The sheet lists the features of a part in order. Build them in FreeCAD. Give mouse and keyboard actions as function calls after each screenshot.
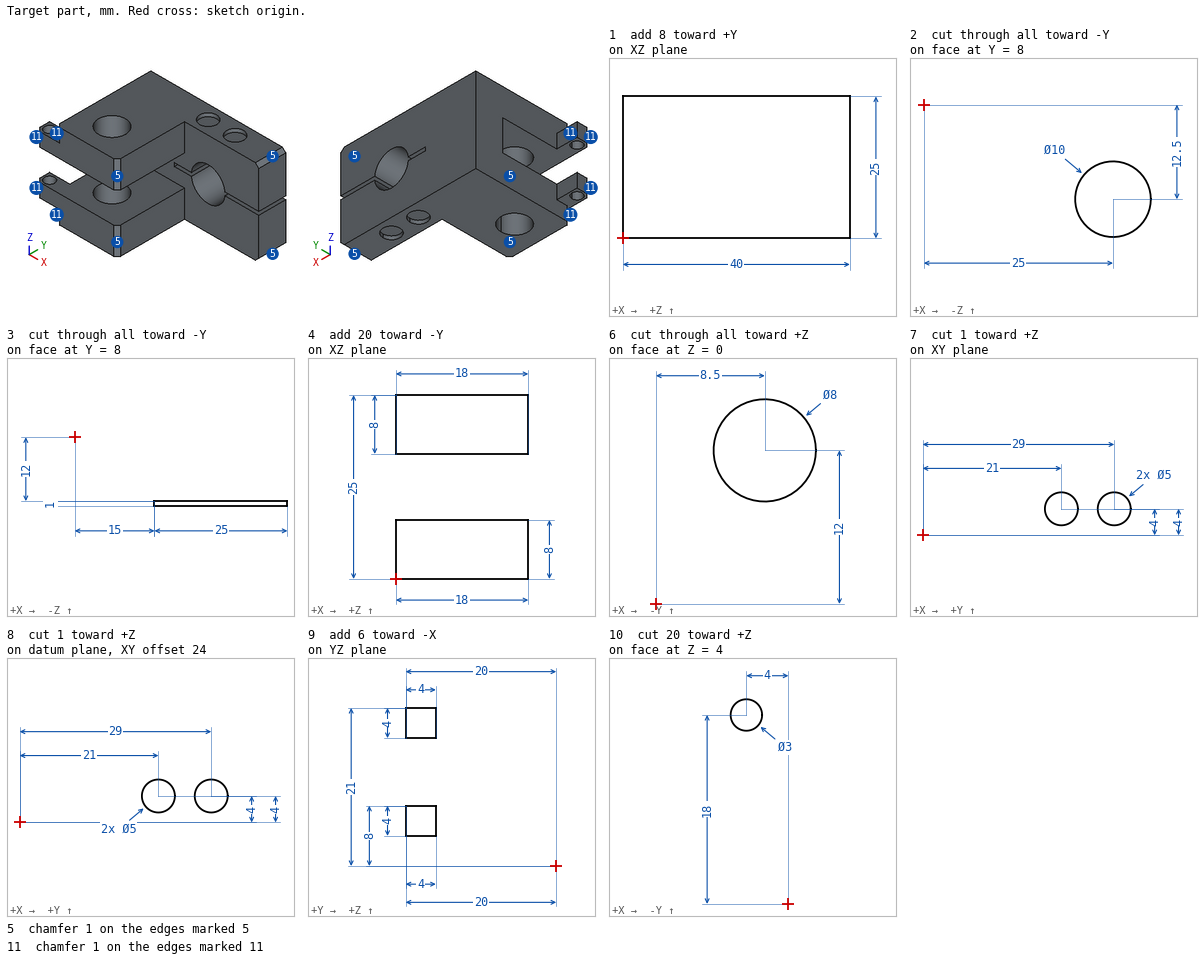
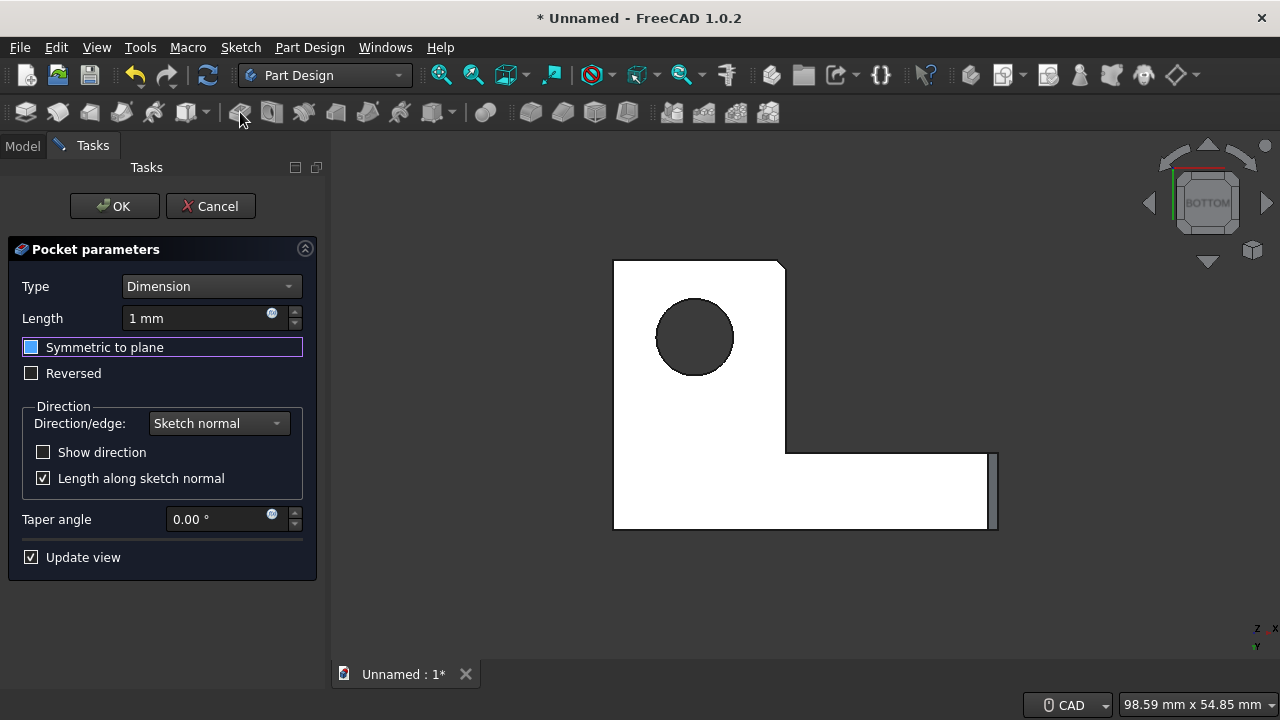
click(30, 373)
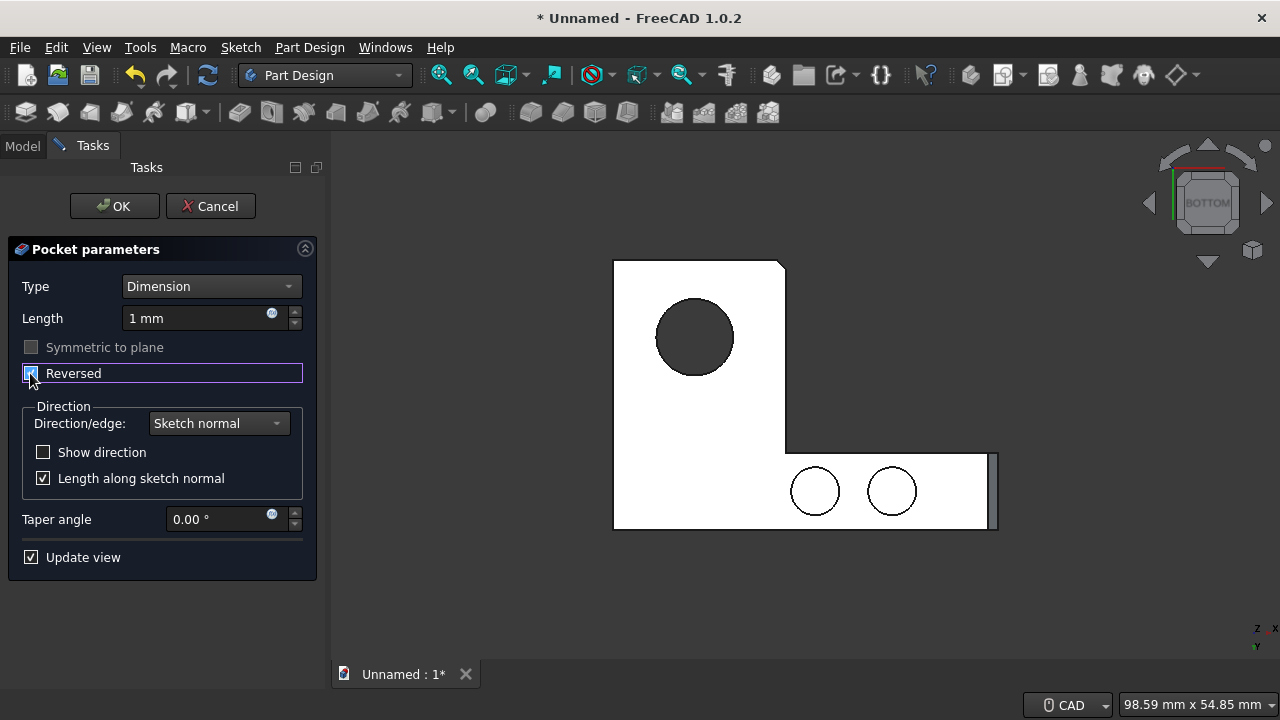
click(115, 206)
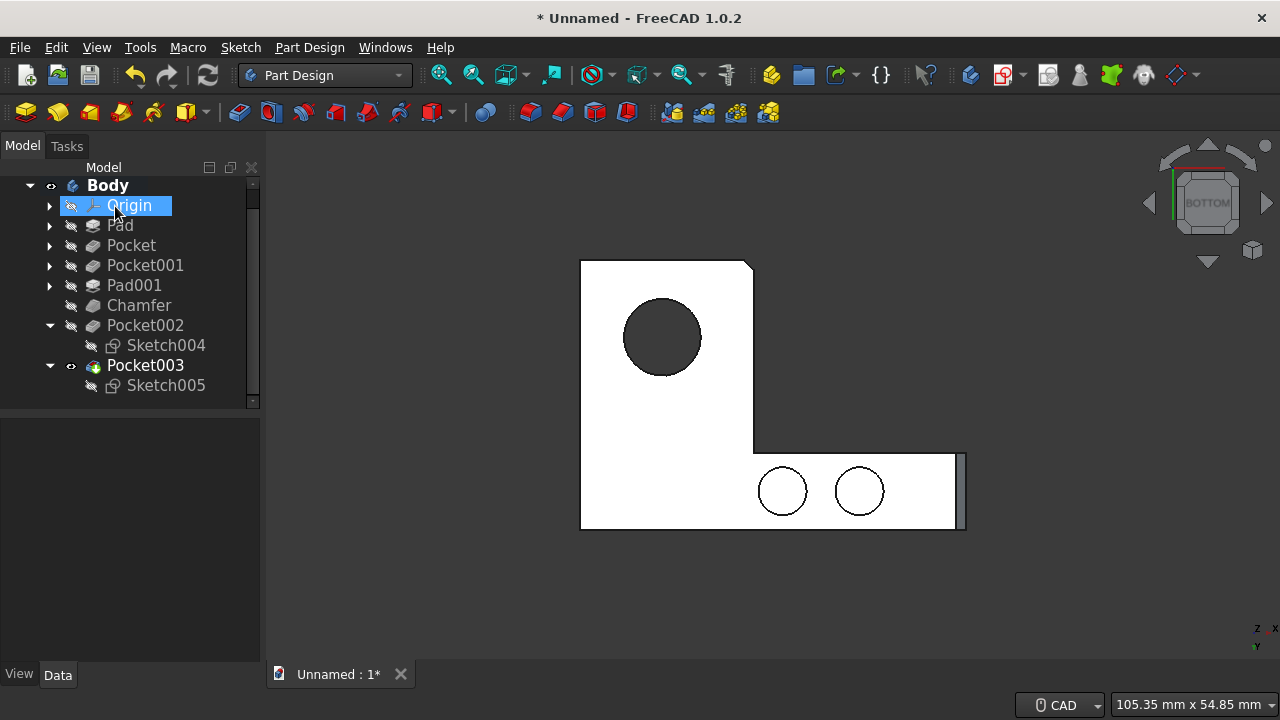
click(50, 206)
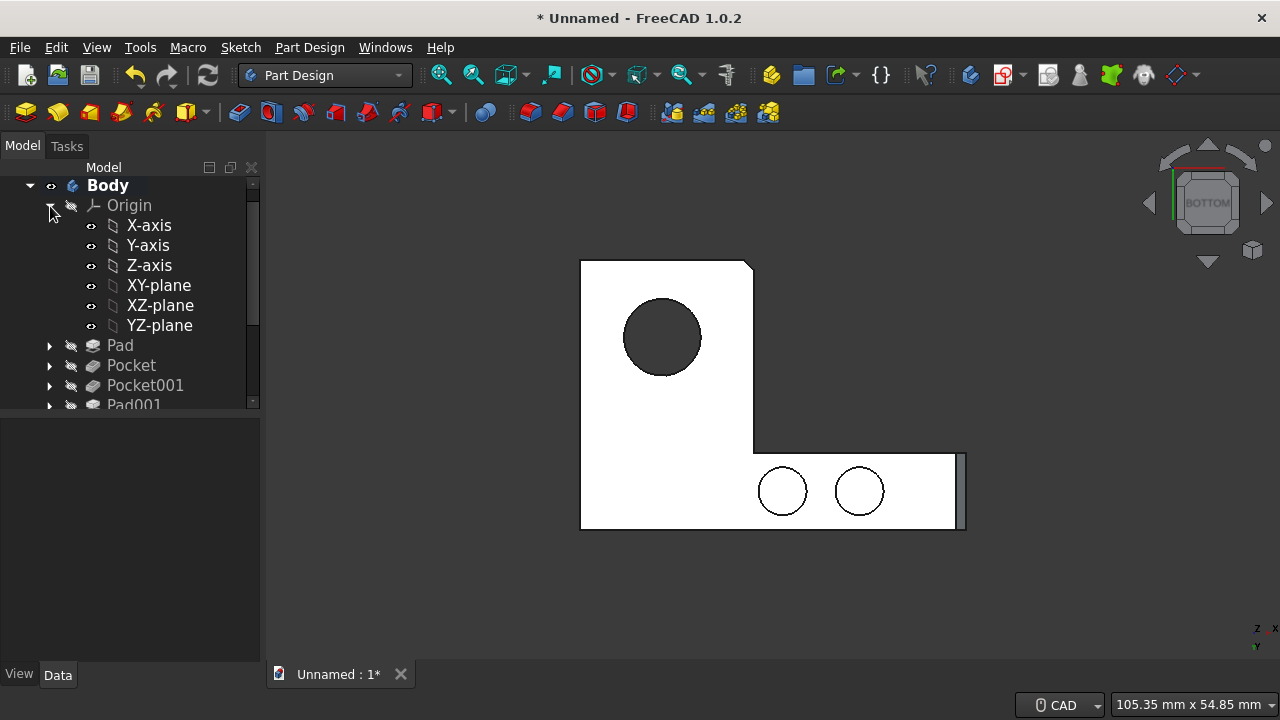
click(136, 286)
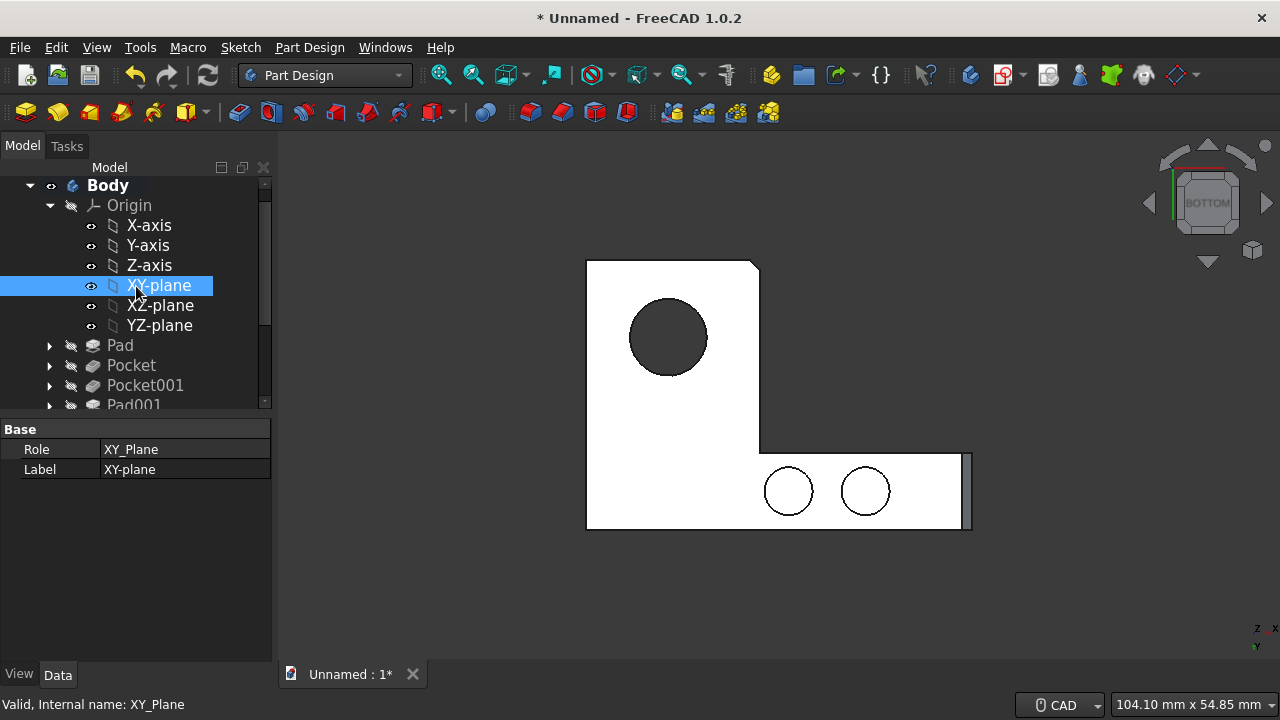
click(1176, 76)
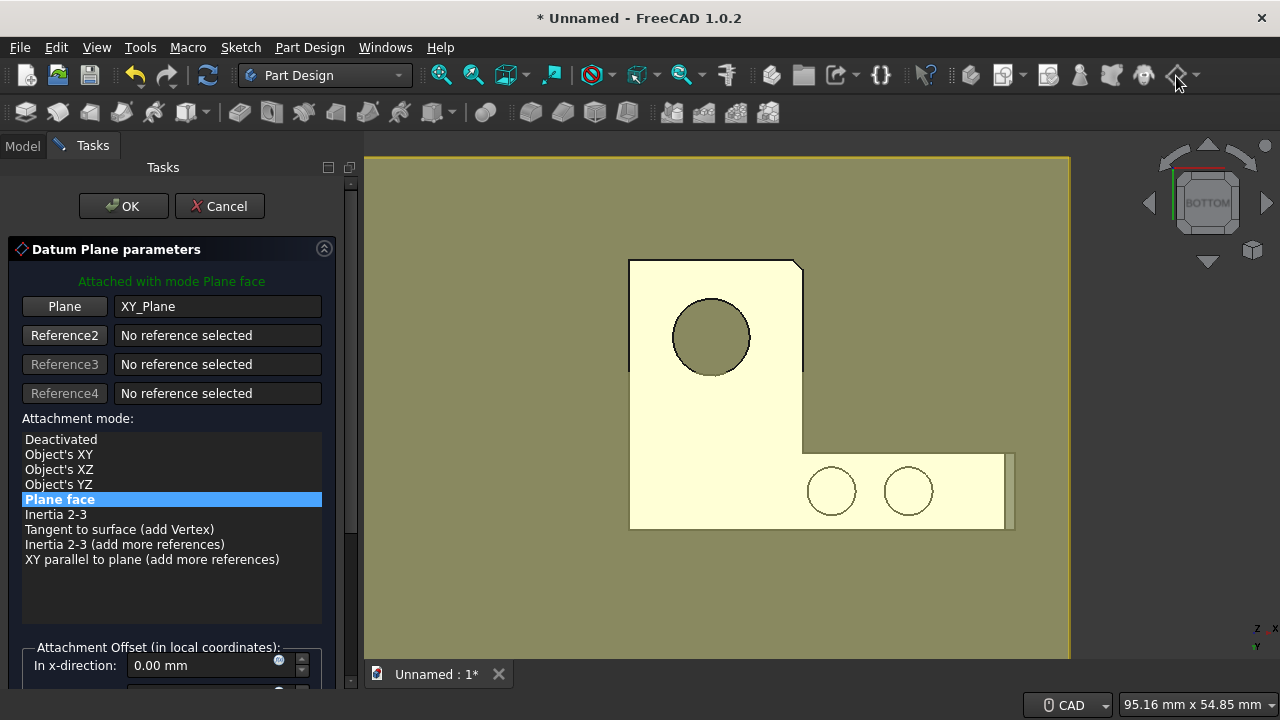
scroll(351, 432, down, 2)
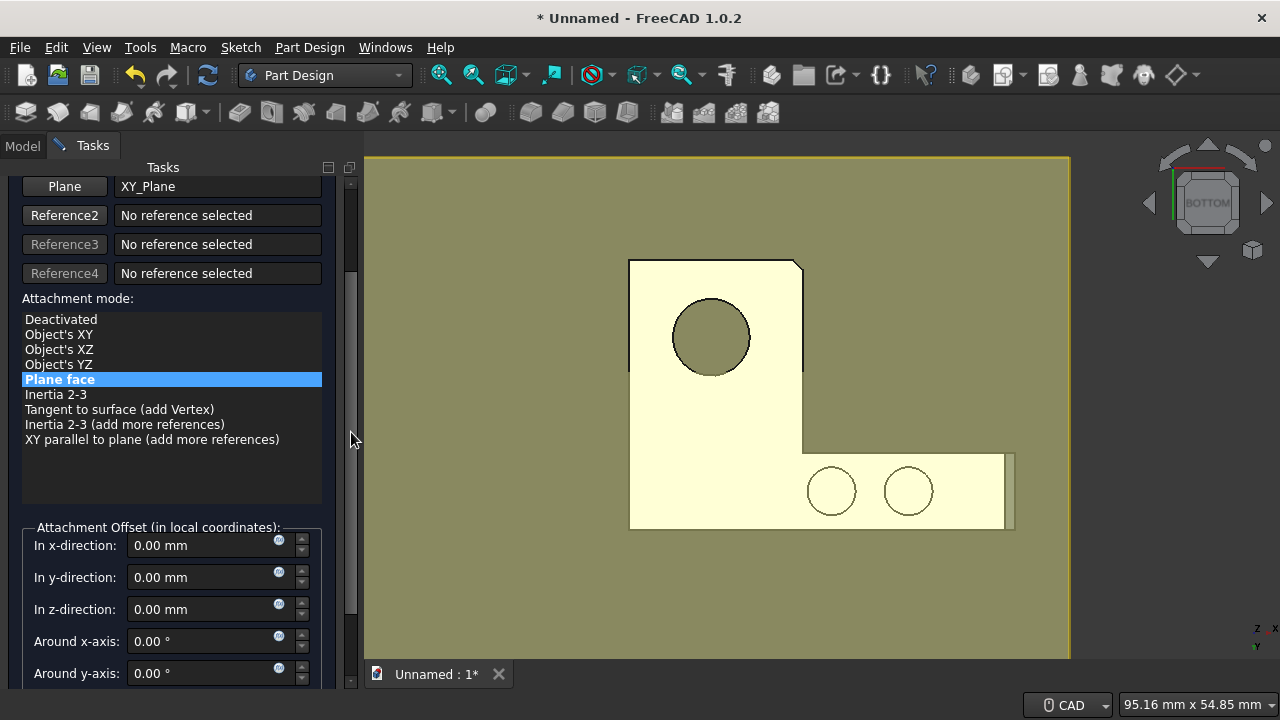
triple_click(210, 609)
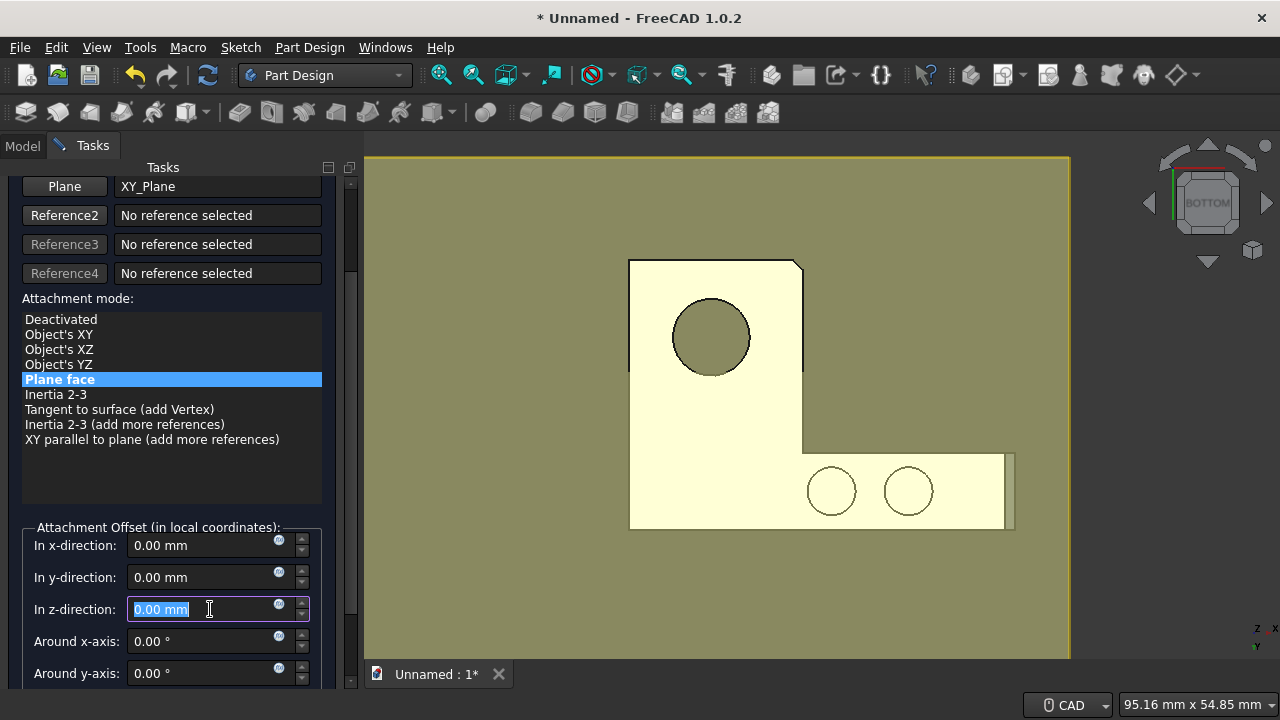
text(24)
key(Tab)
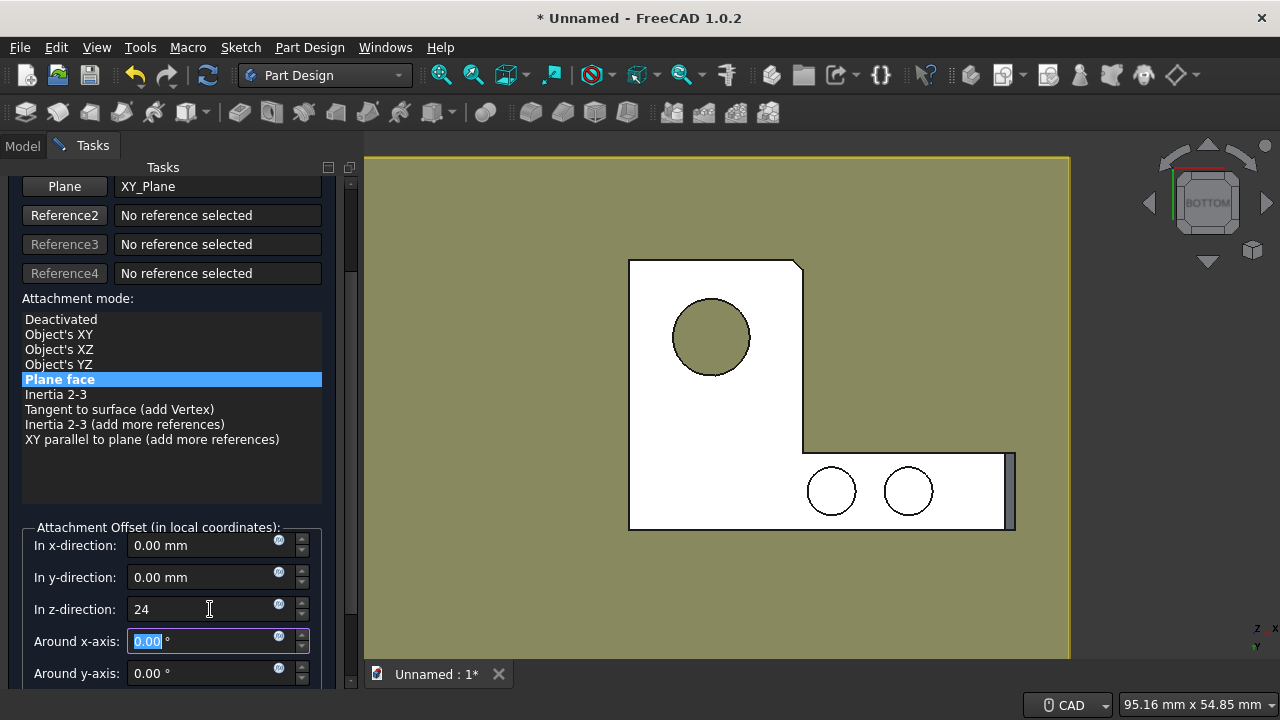
scroll(351, 432, up, 3)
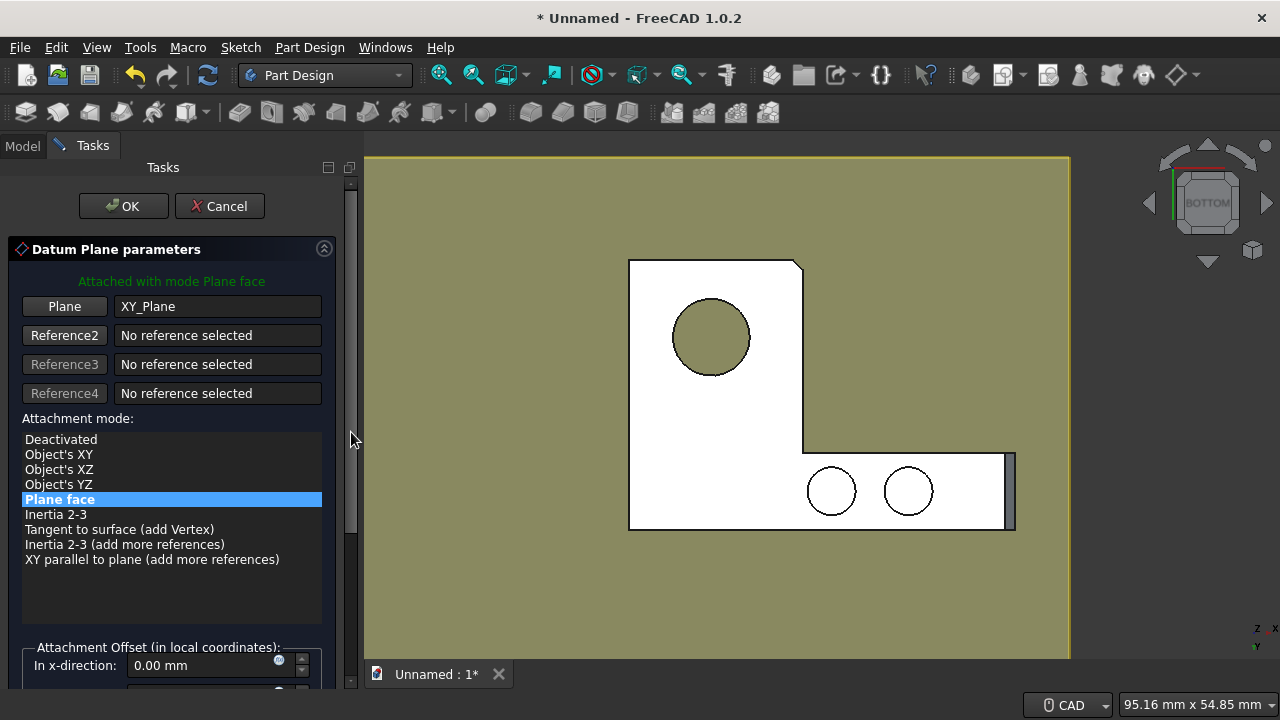
click(124, 206)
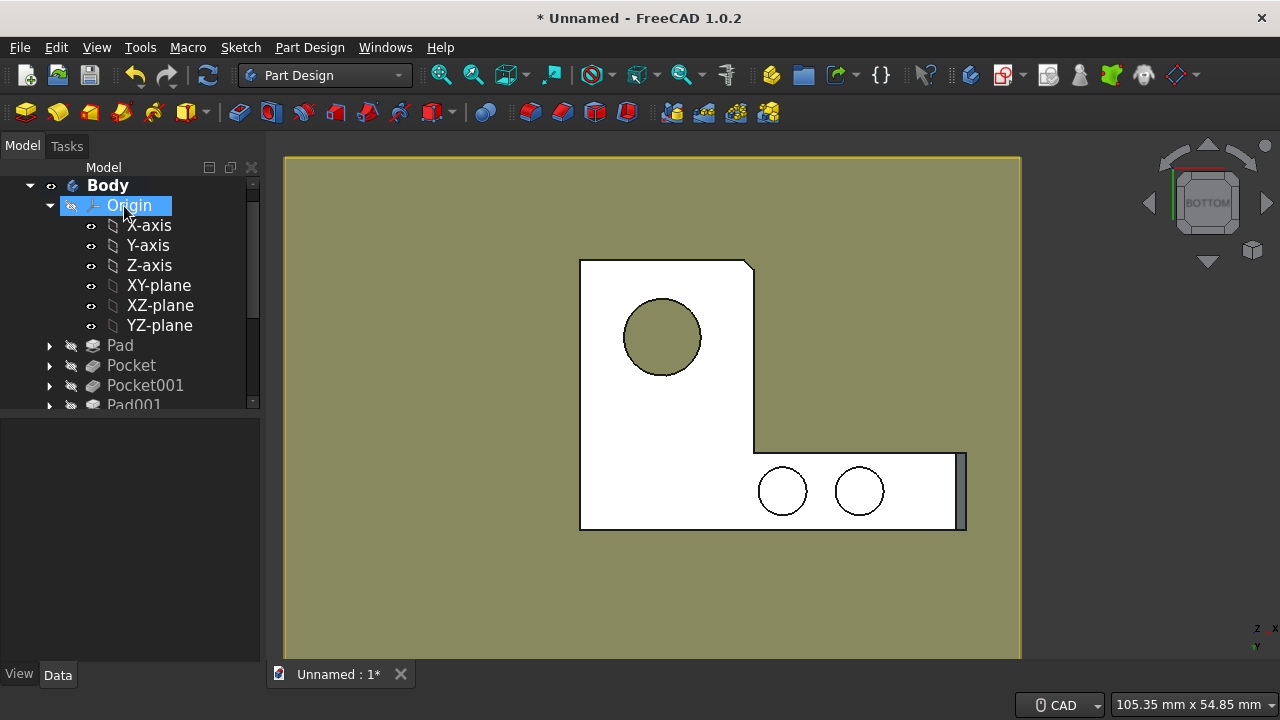
scroll(120, 301, down, 3)